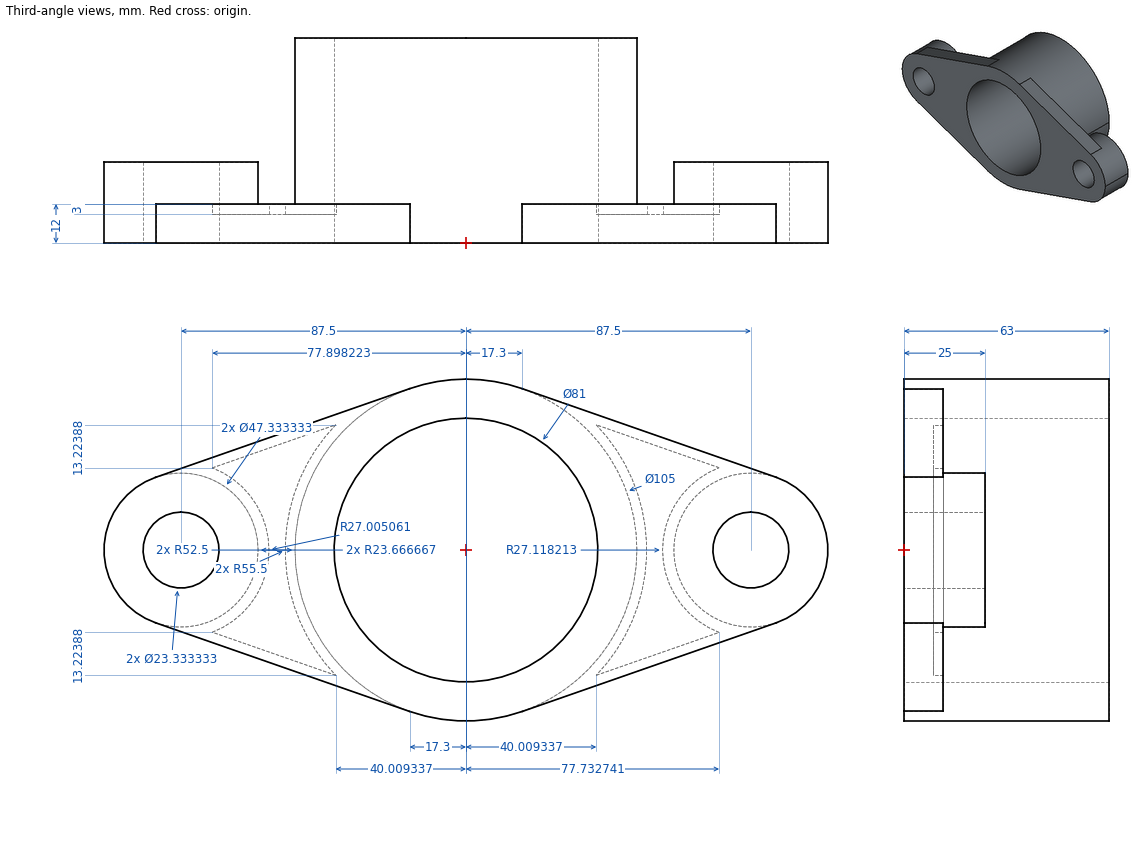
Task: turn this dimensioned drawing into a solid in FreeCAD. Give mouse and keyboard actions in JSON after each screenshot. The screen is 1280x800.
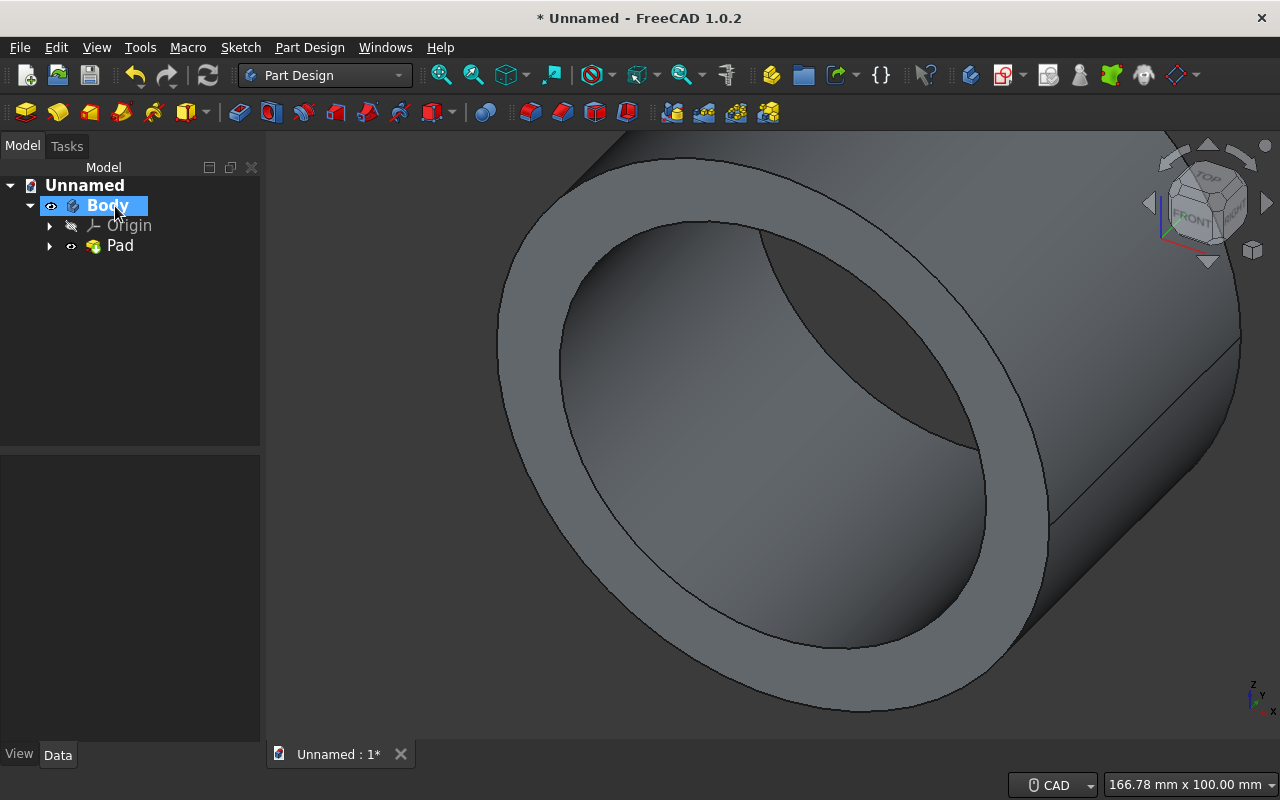
{"action": "key", "text": "v f"}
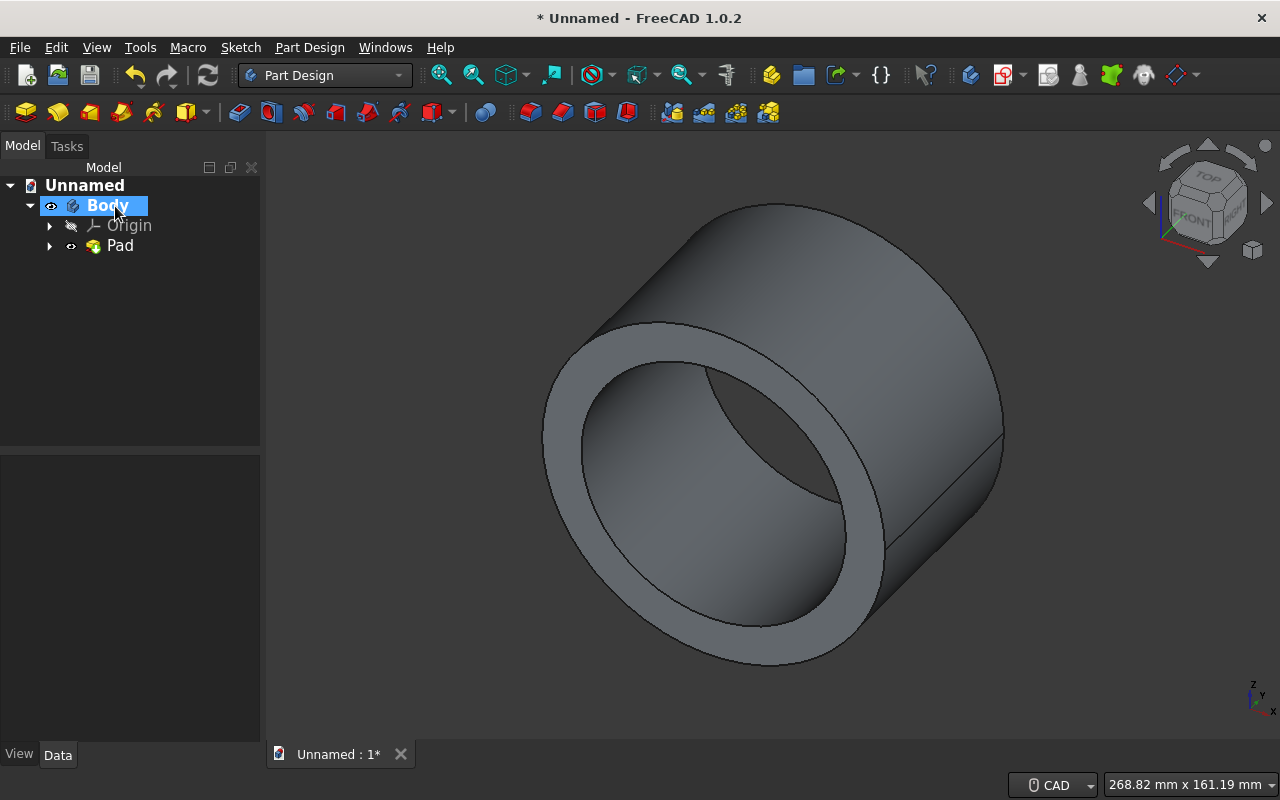
{"action": "left_click", "coordinate": [1004, 76]}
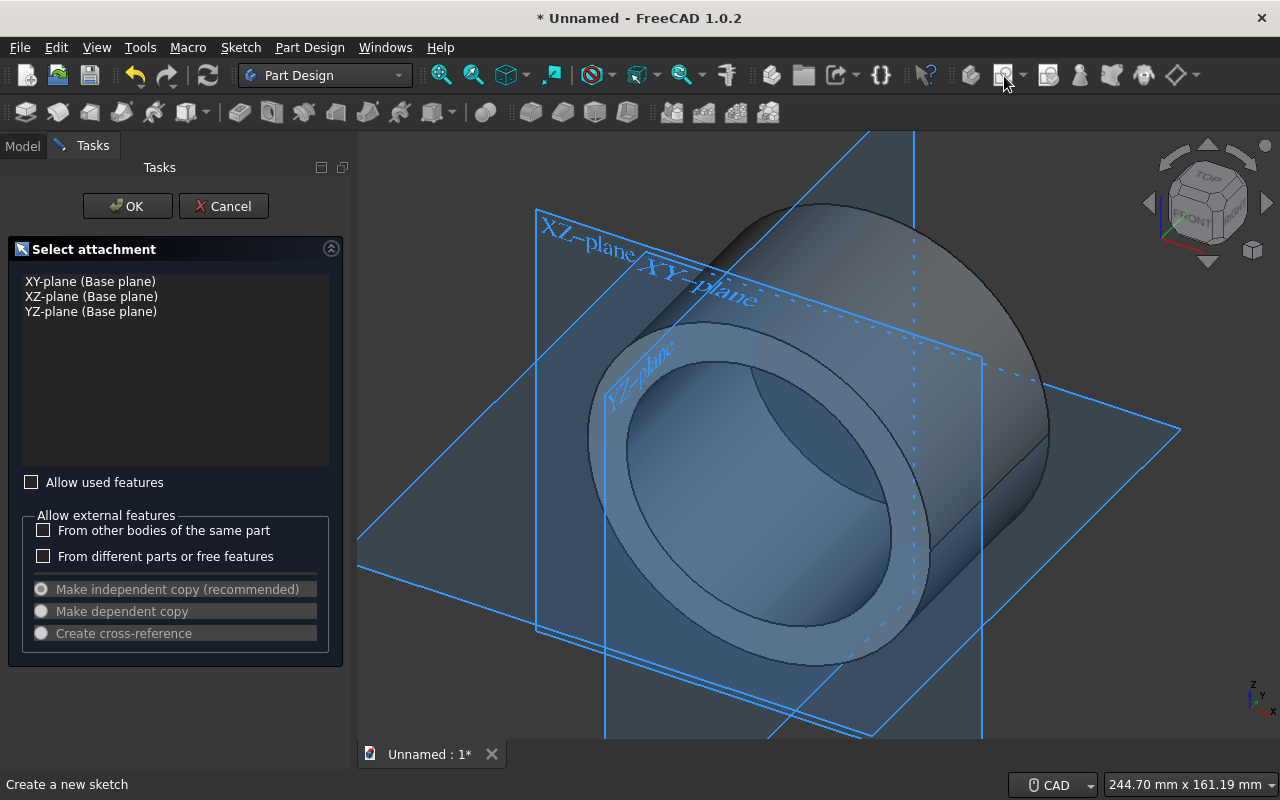
{"action": "left_click", "coordinate": [82, 296]}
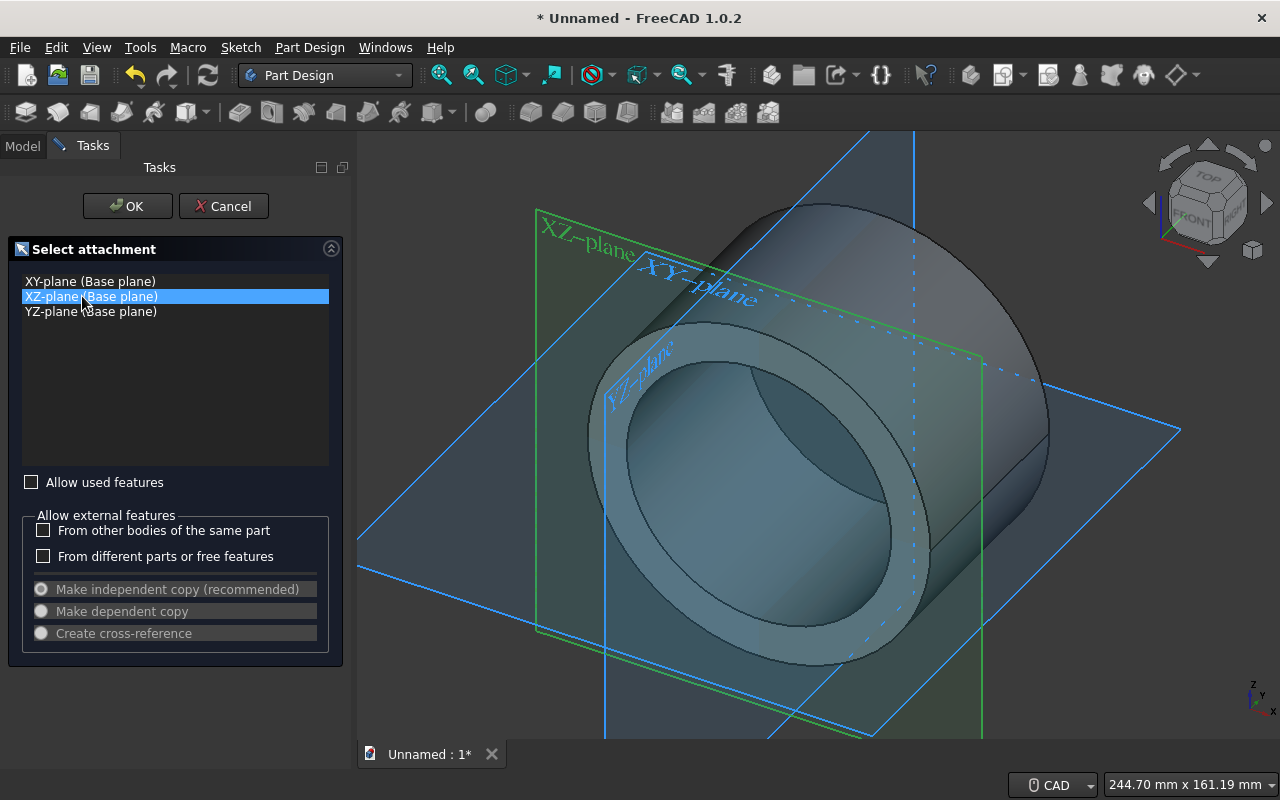
{"action": "left_click", "coordinate": [128, 206]}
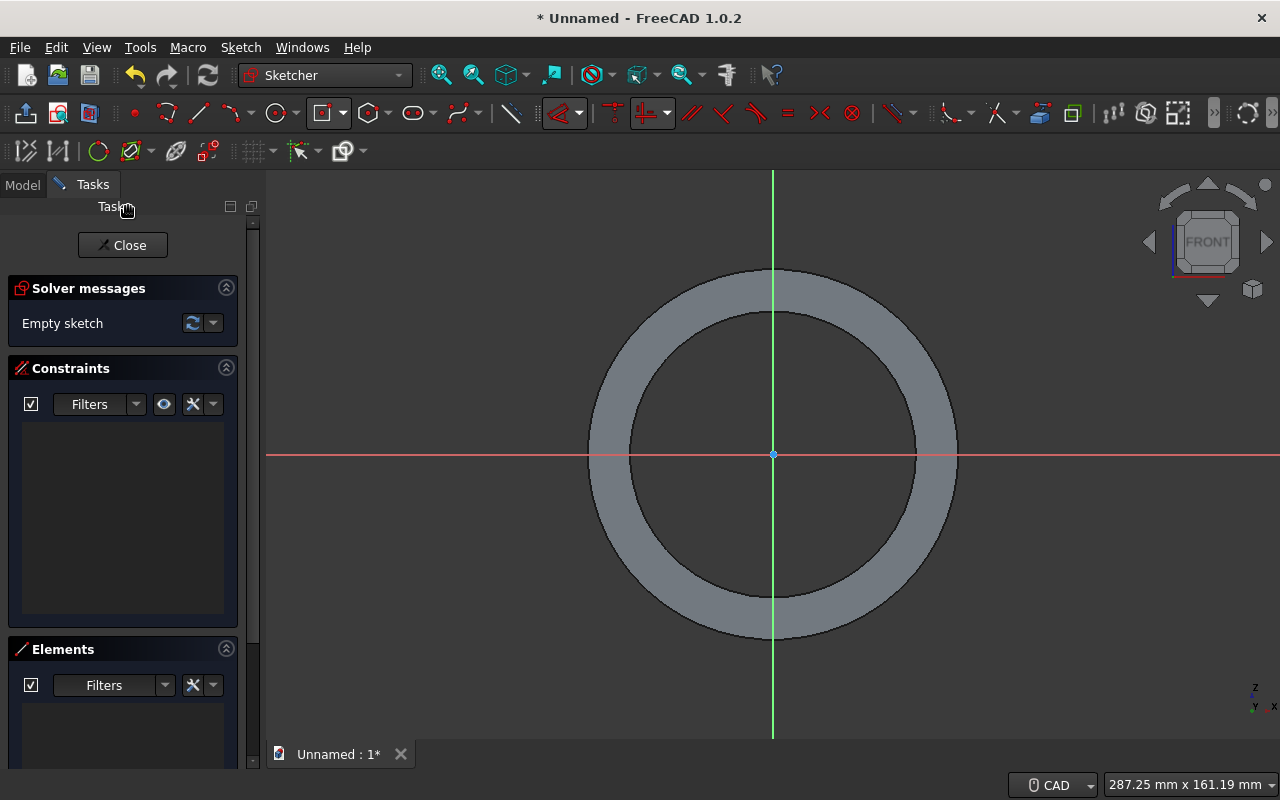
{"action": "scroll", "coordinate": [395, 454], "scroll_direction": "down", "scroll_amount": 1}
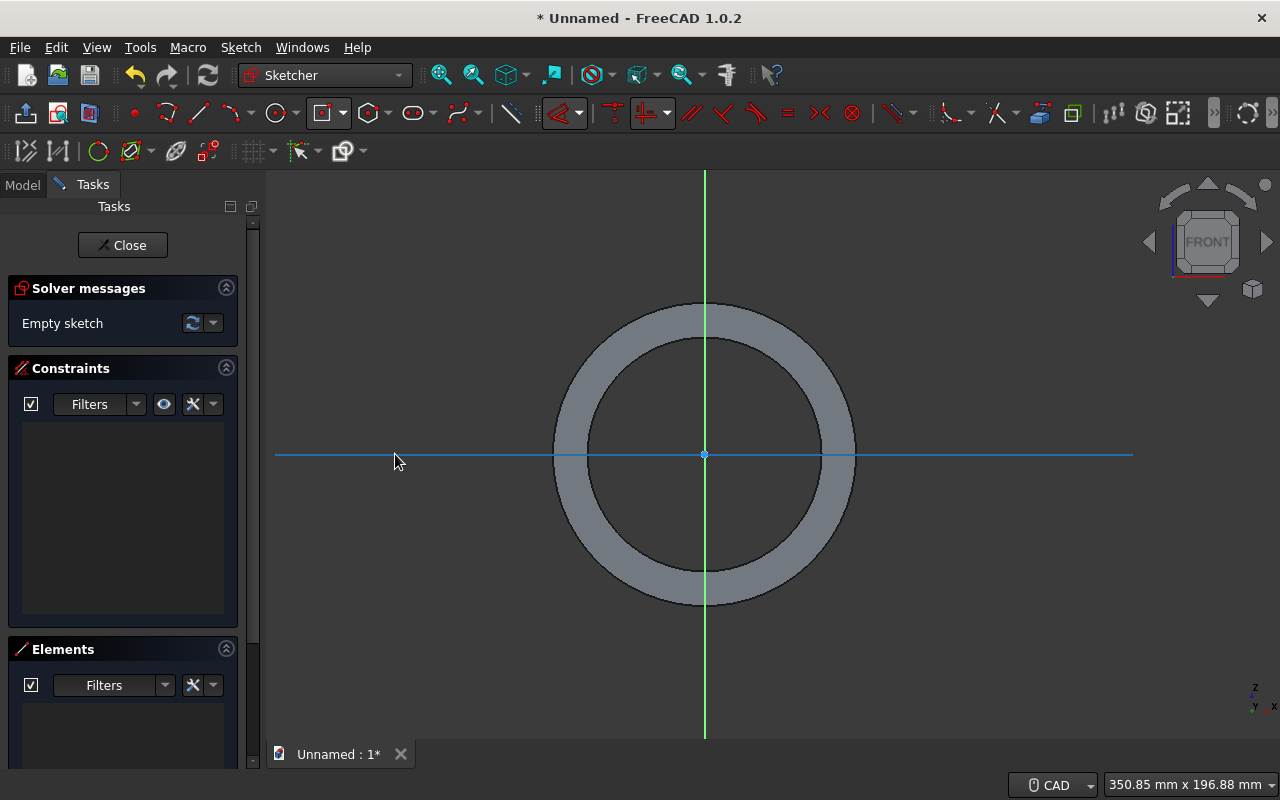
{"action": "key", "text": "g l"}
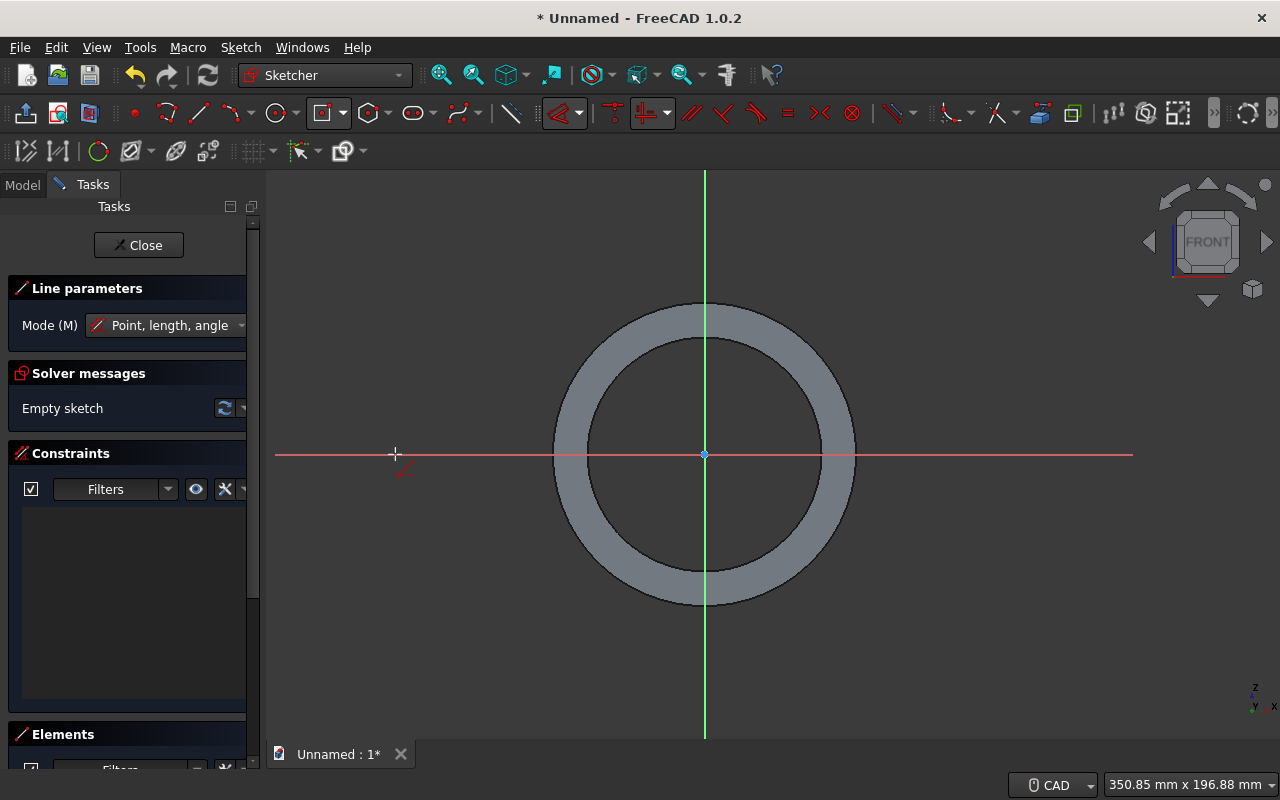
{"action": "left_click", "coordinate": [655, 598]}
{"action": "left_click", "coordinate": [429, 519]}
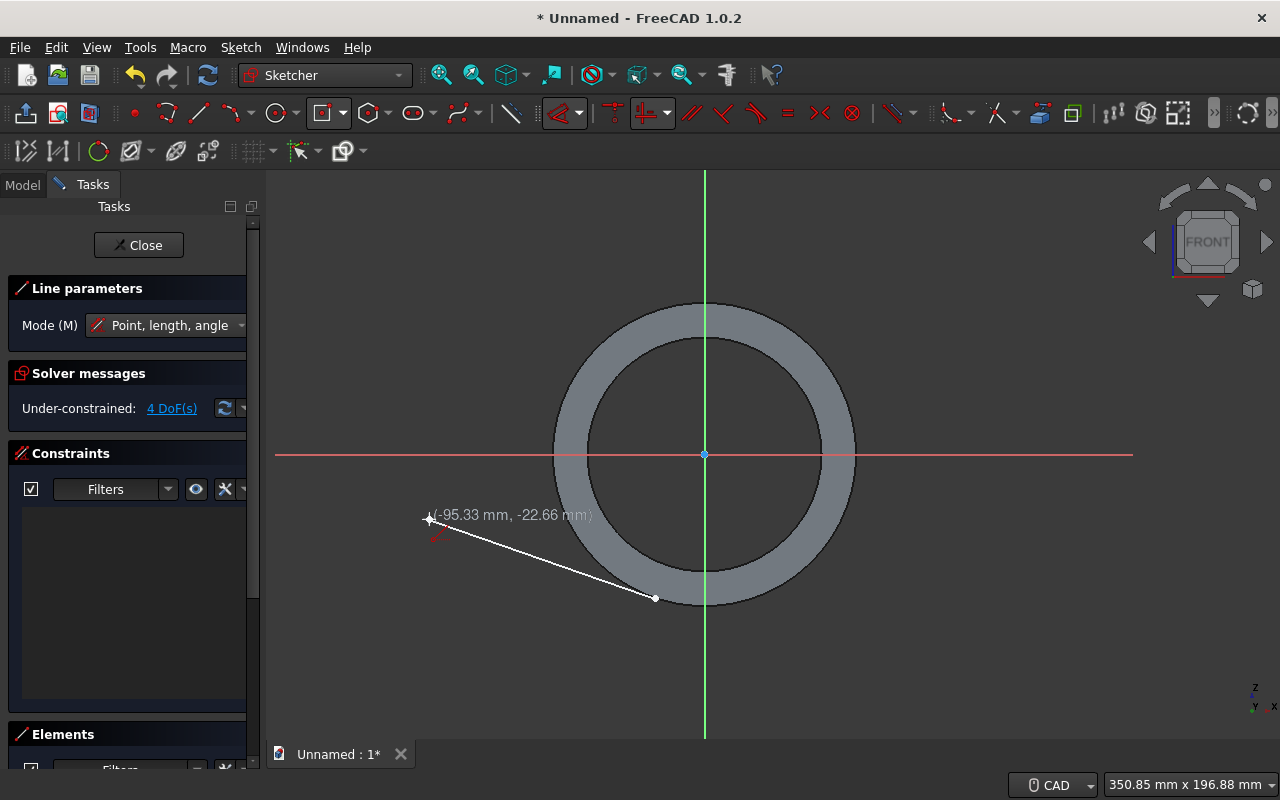
{"action": "left_click", "coordinate": [429, 390]}
{"action": "left_click", "coordinate": [655, 311]}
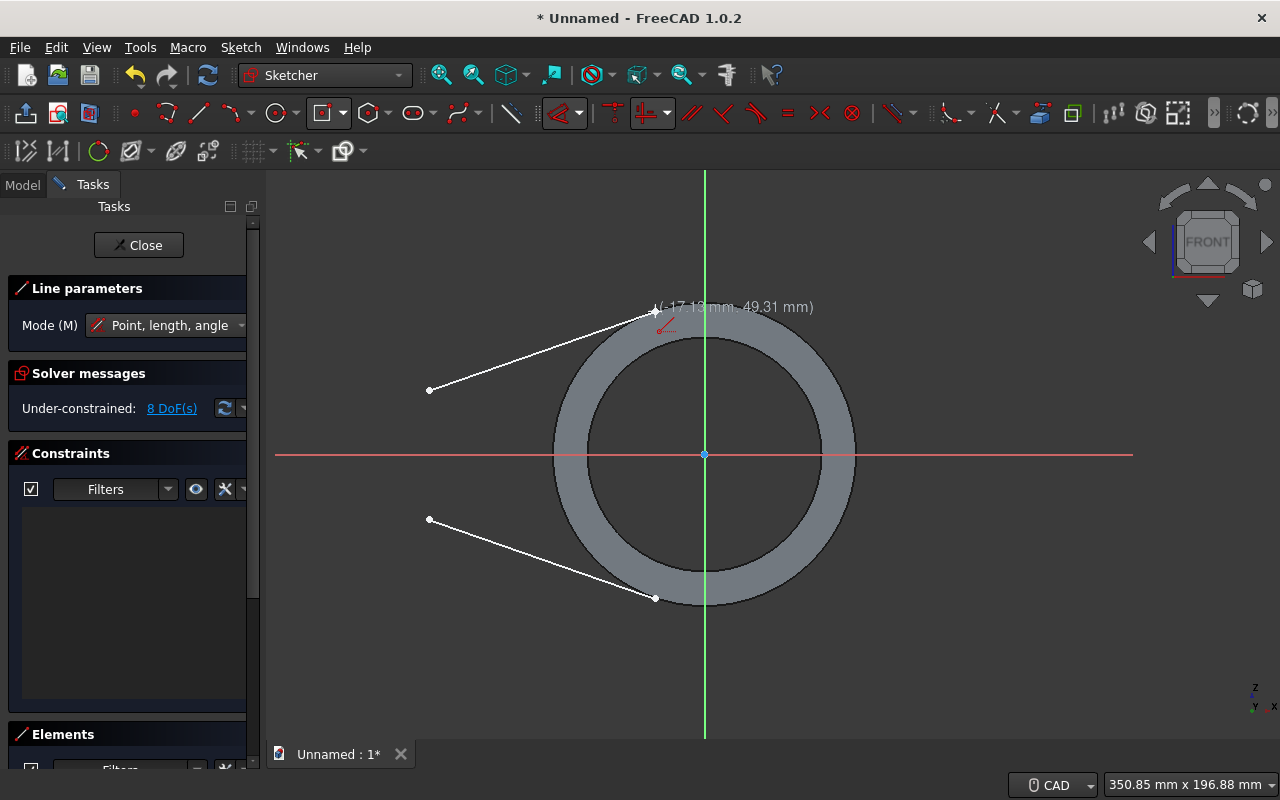
{"action": "left_click", "coordinate": [232, 114]}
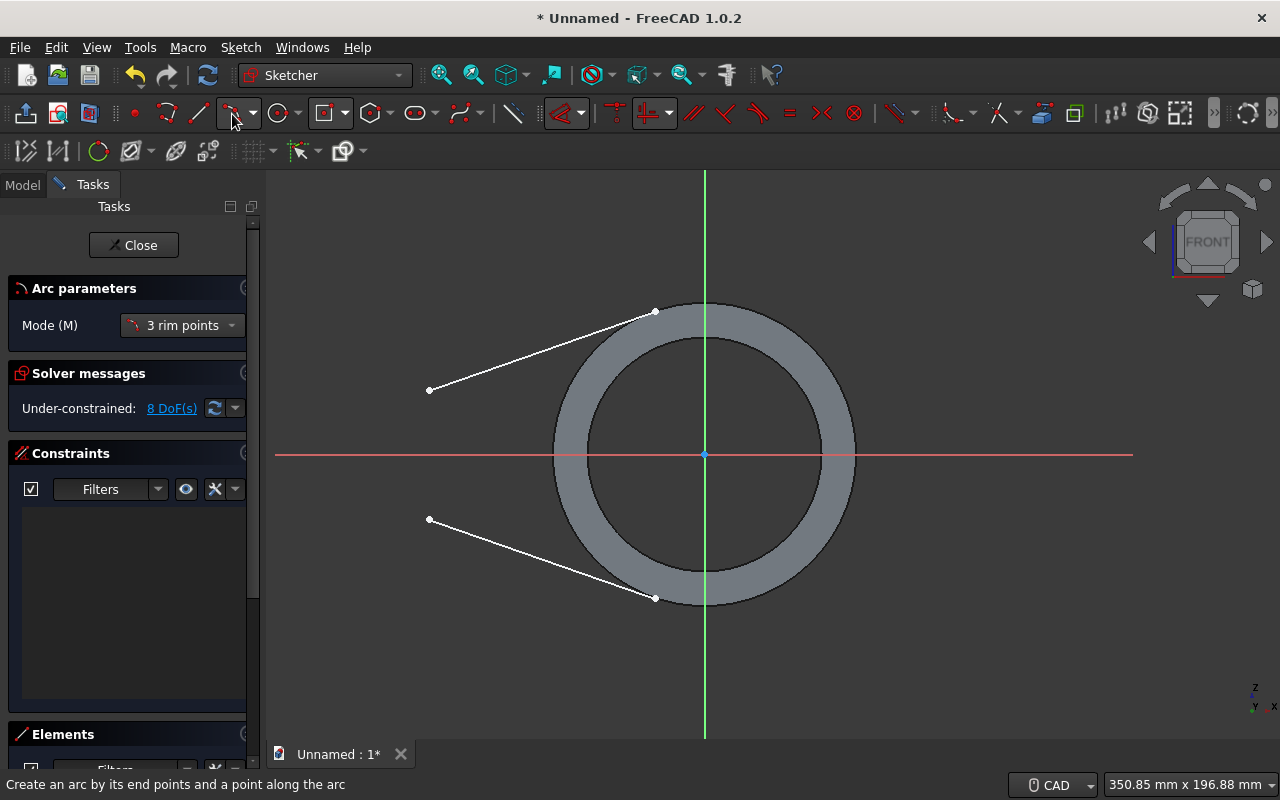
{"action": "left_click", "coordinate": [429, 520]}
{"action": "left_click", "coordinate": [429, 391]}
{"action": "left_click", "coordinate": [515, 480]}